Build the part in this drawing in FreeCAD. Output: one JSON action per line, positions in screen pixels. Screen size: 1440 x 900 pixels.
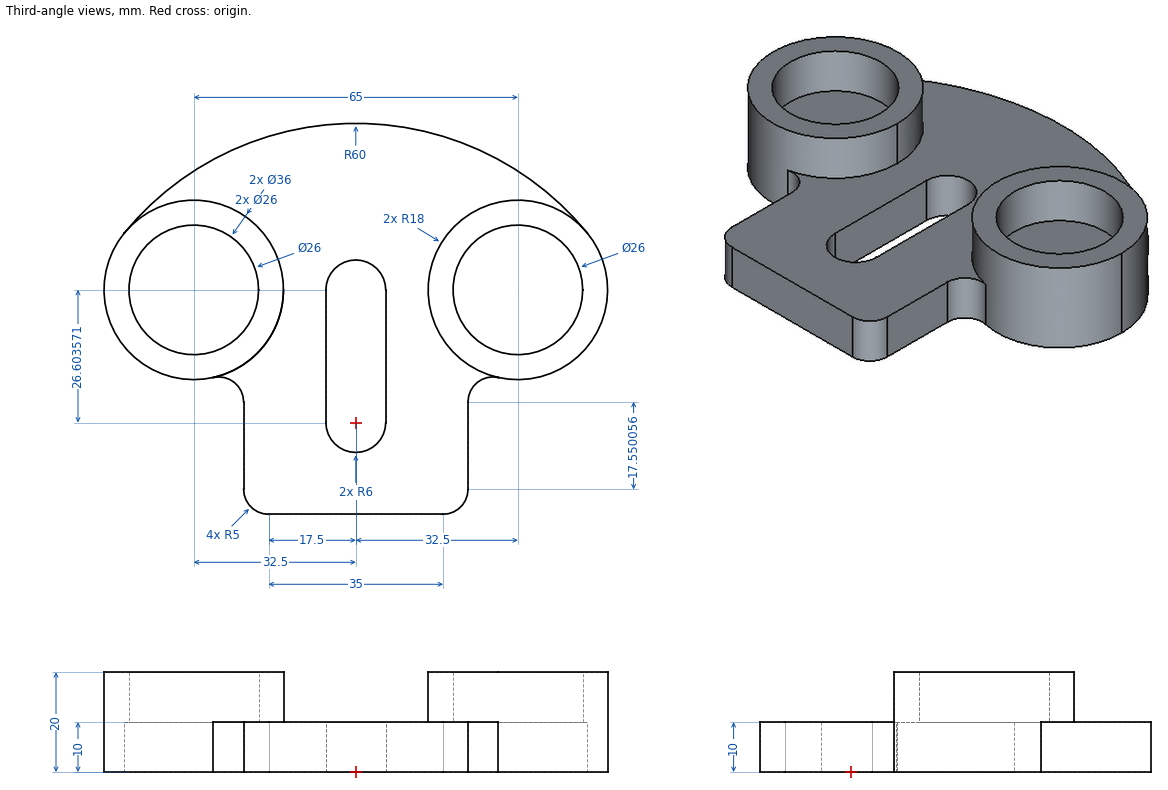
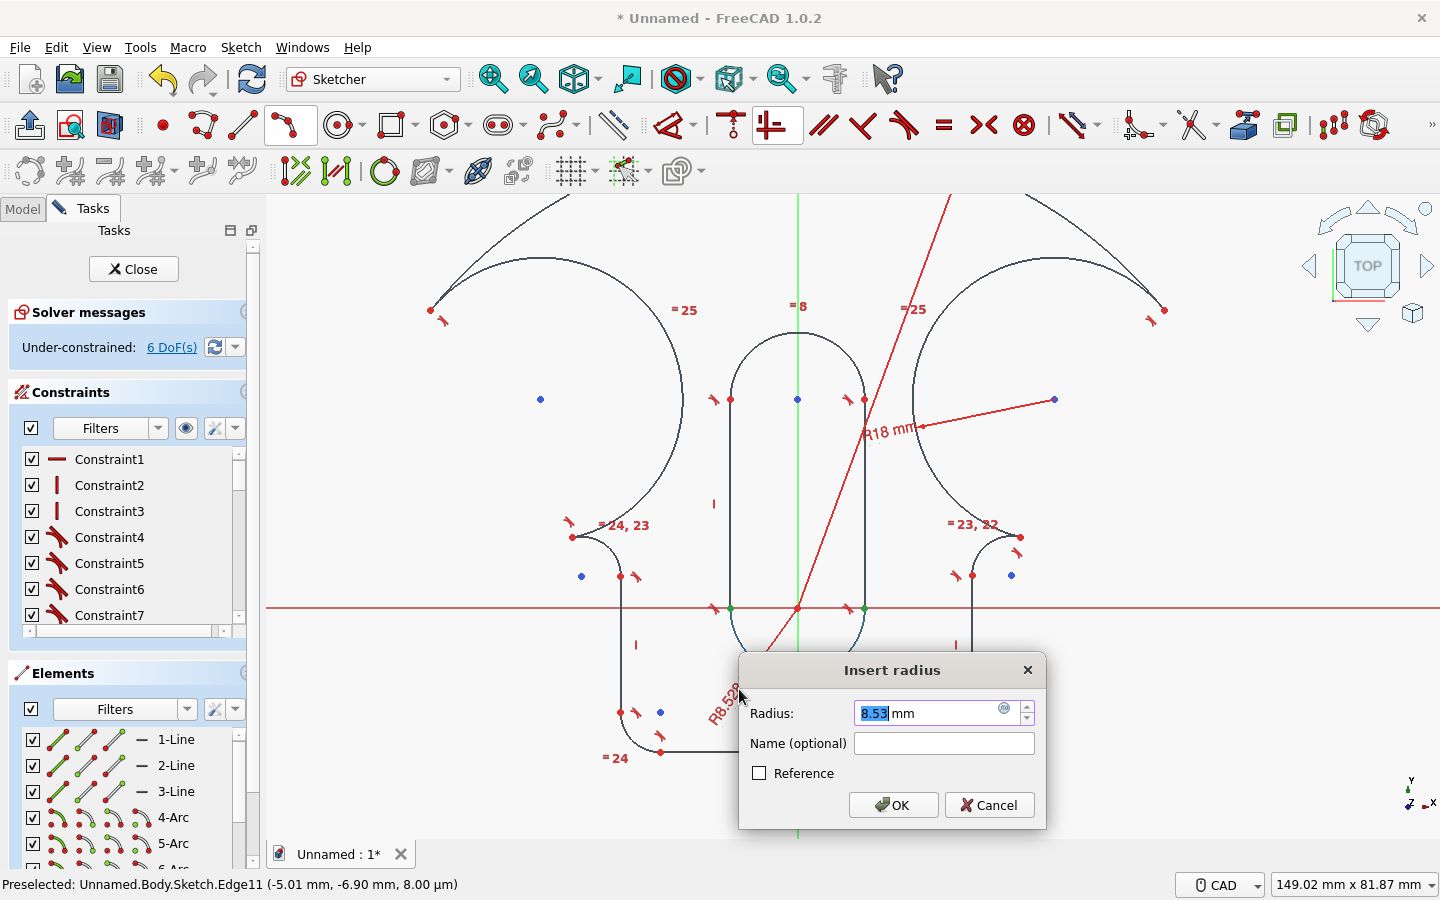
{"action": "type", "text": "6"}
{"action": "key", "text": "Return"}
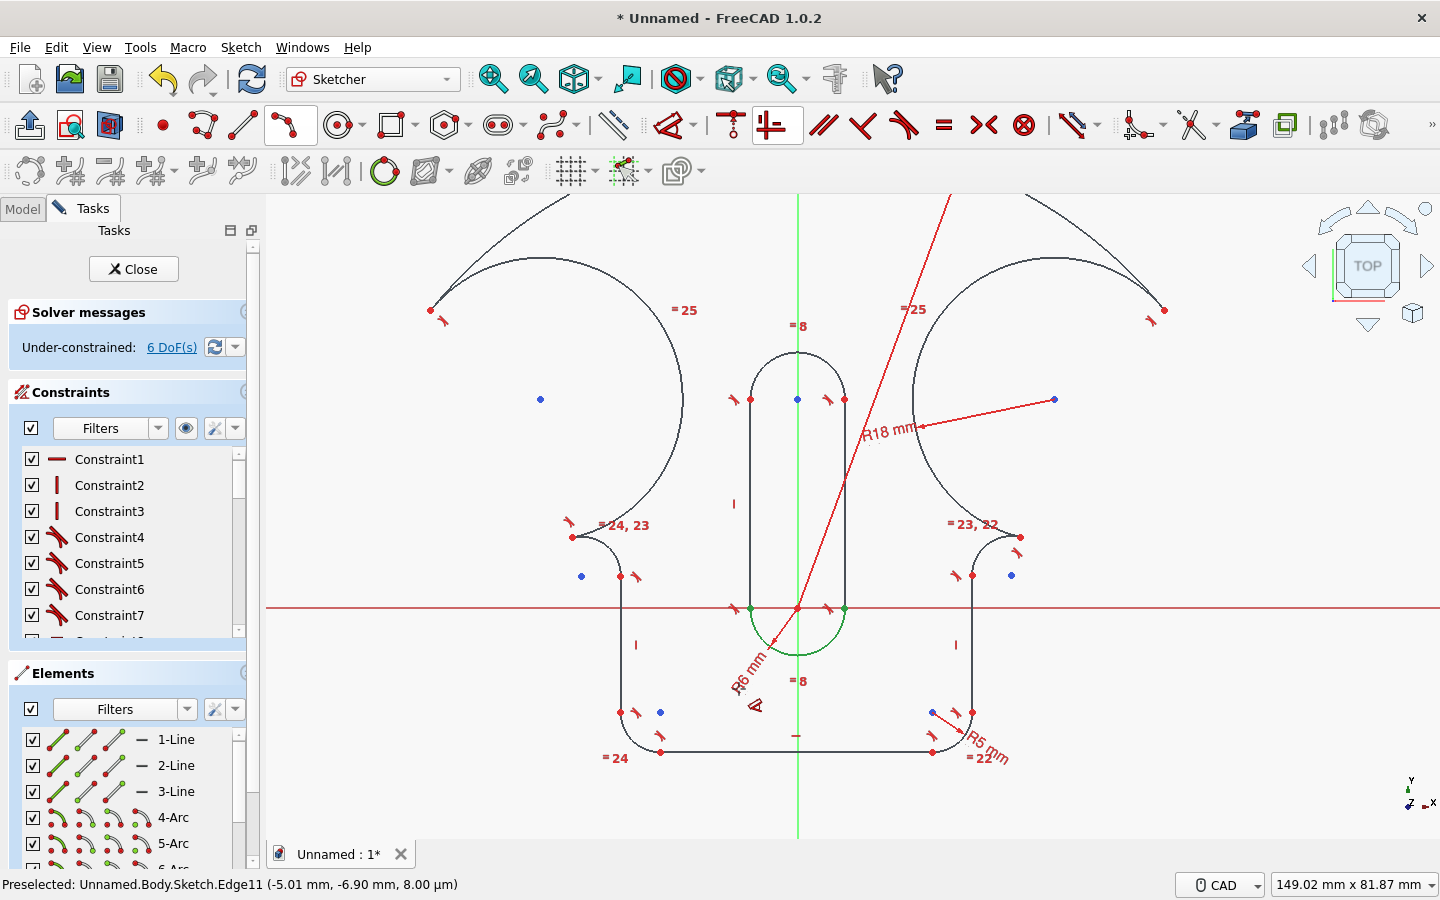
{"action": "left_click", "coordinate": [742, 752]}
{"action": "left_click", "coordinate": [734, 786]}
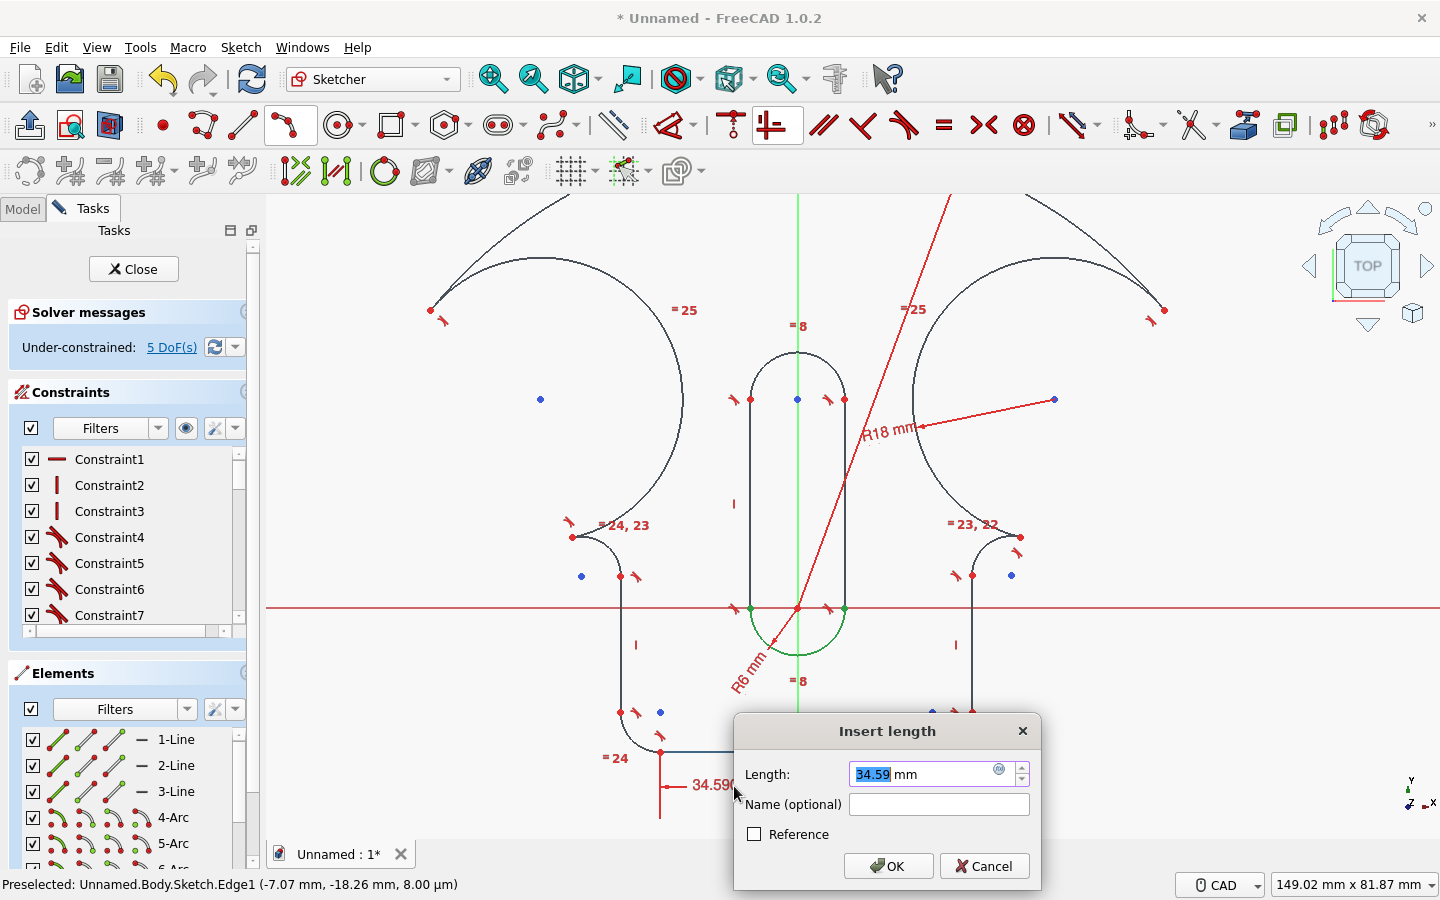
{"action": "type", "text": "35"}
{"action": "key", "text": "Return"}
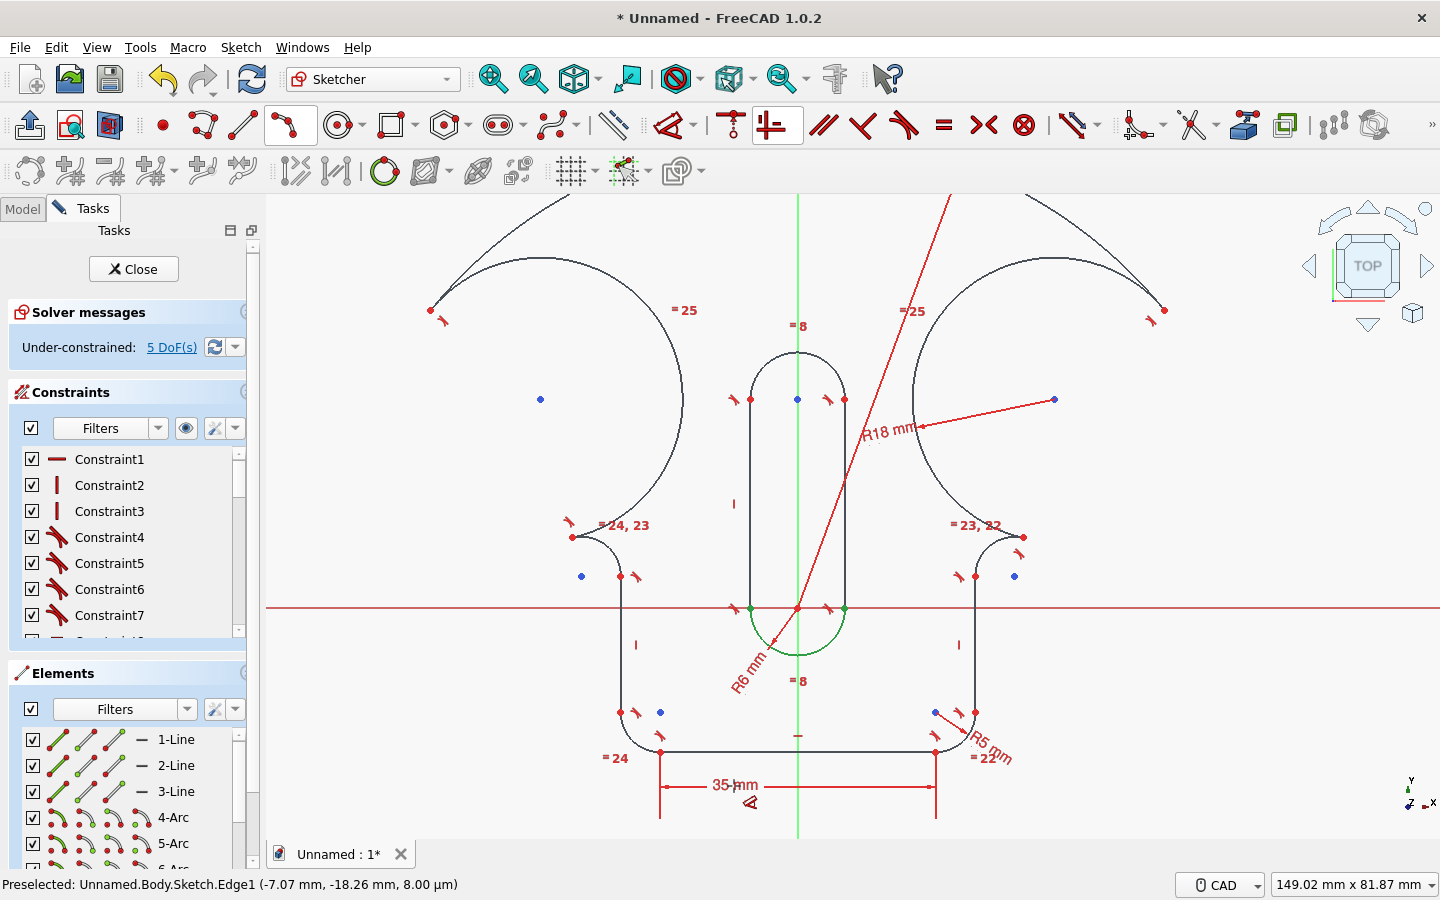
{"action": "left_click", "coordinate": [660, 752]}
{"action": "left_click", "coordinate": [729, 574]}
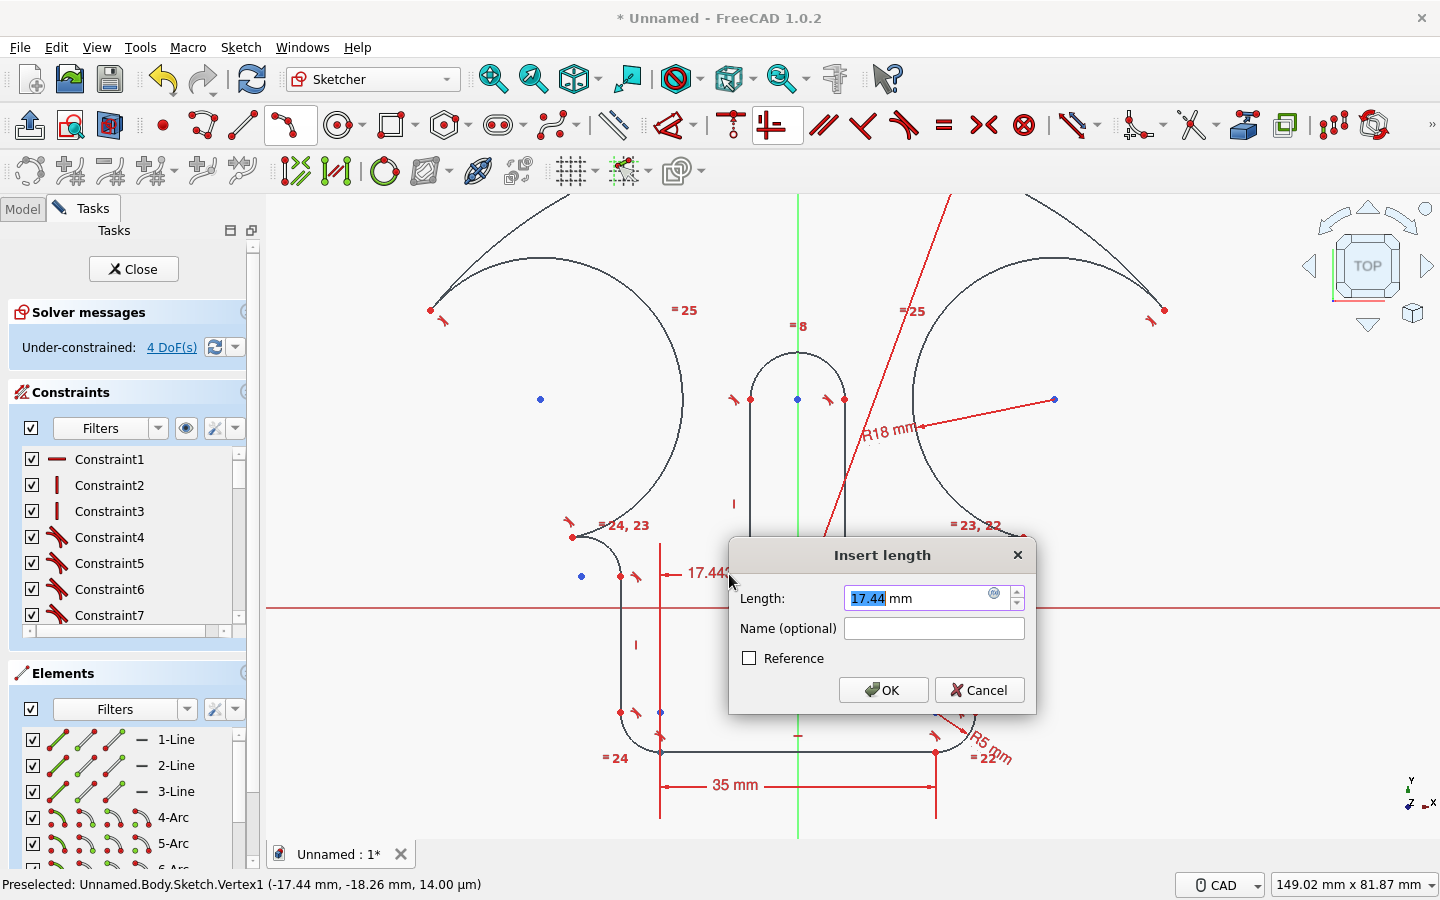
{"action": "type", "text": "17.5"}
{"action": "key", "text": "Return"}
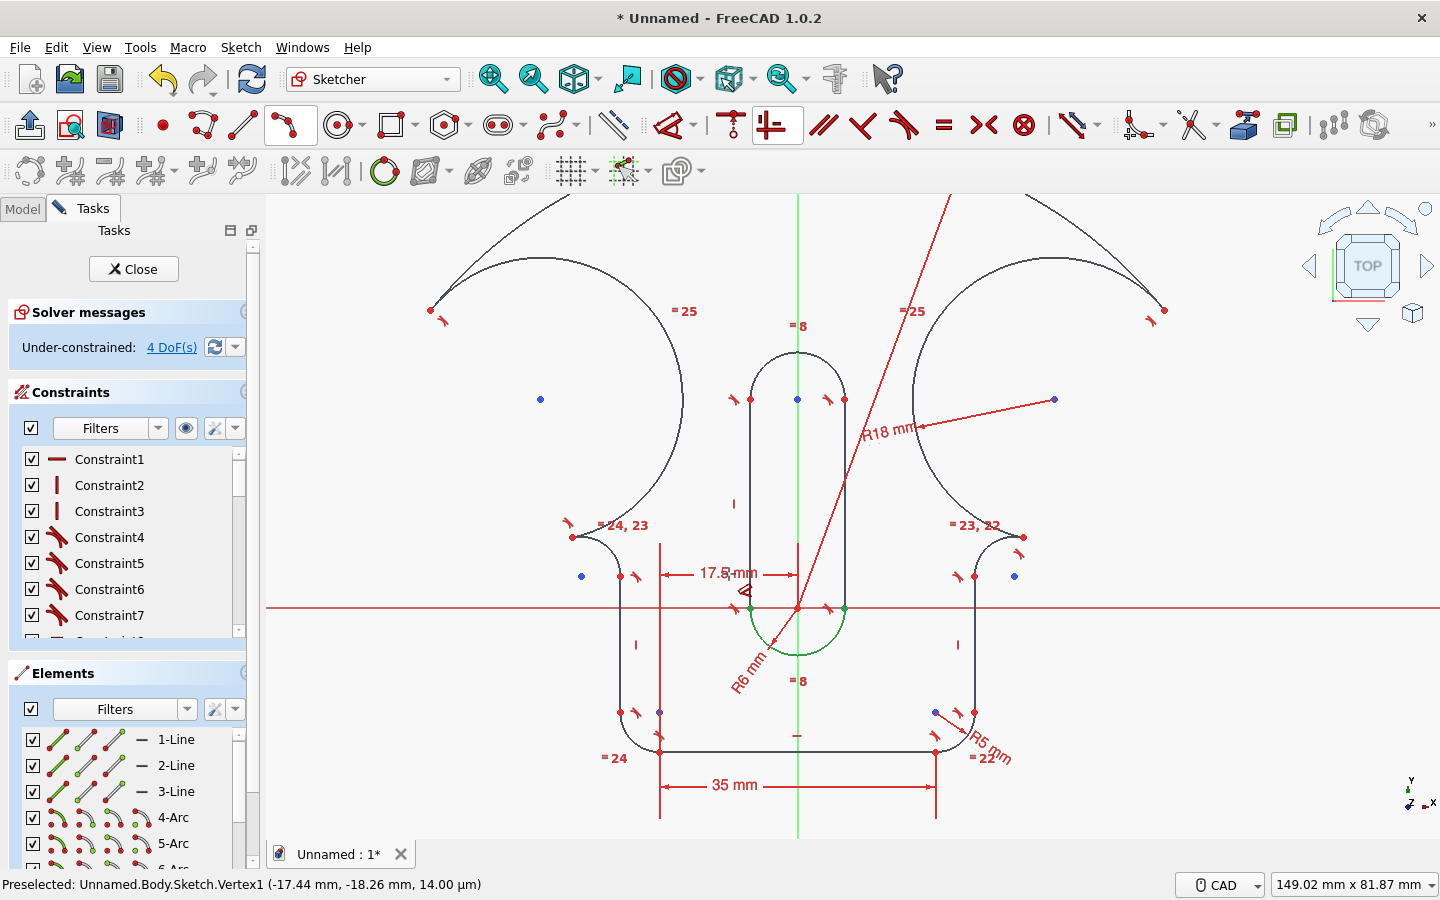
{"action": "left_click", "coordinate": [1054, 399]}
{"action": "left_click", "coordinate": [926, 642]}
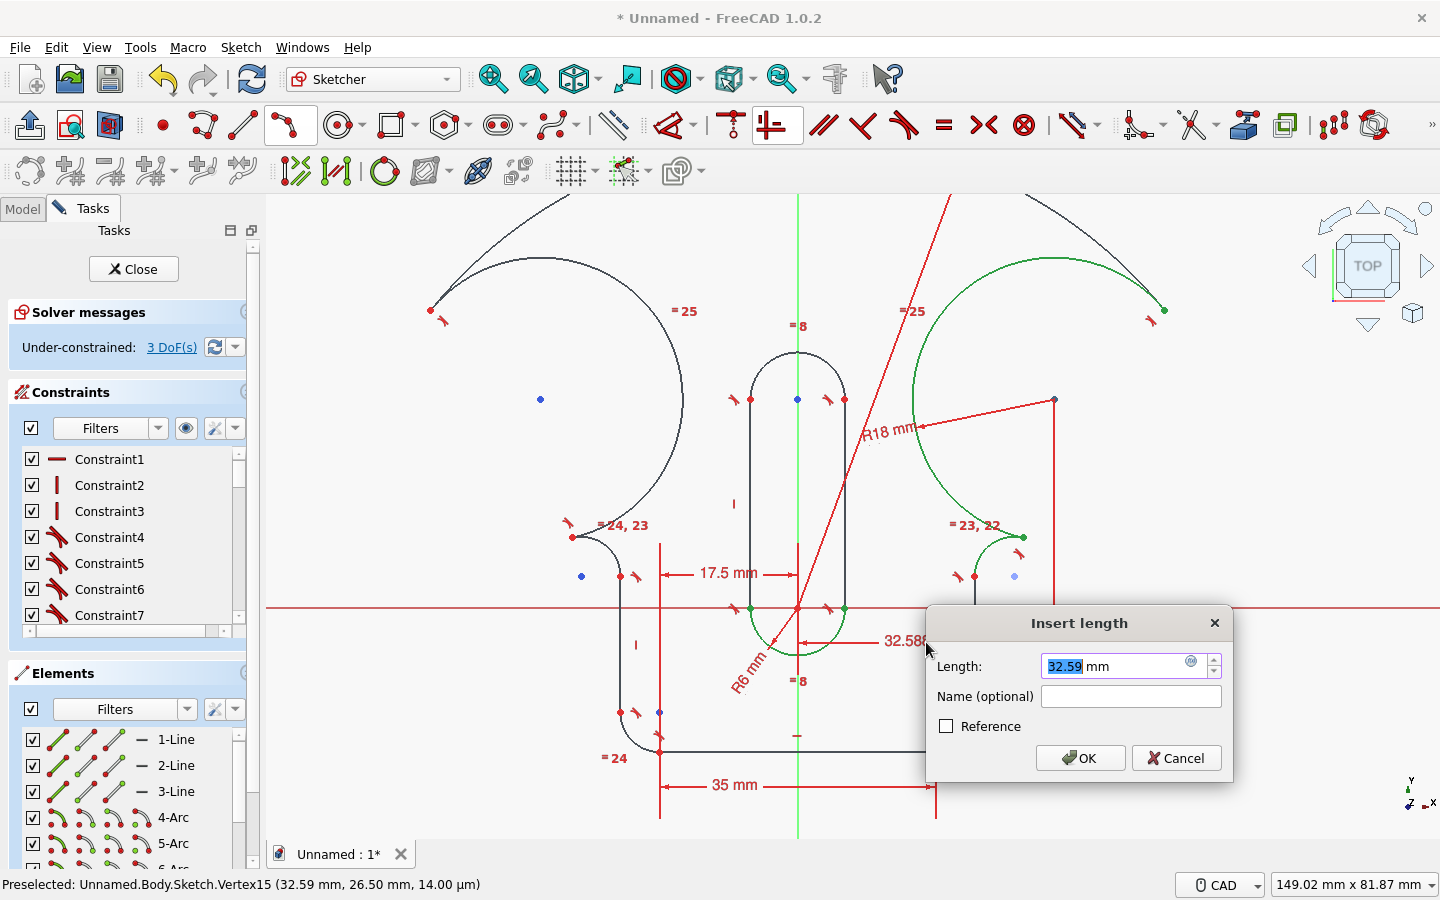
{"action": "type", "text": "32.5"}
{"action": "key", "text": "Return"}